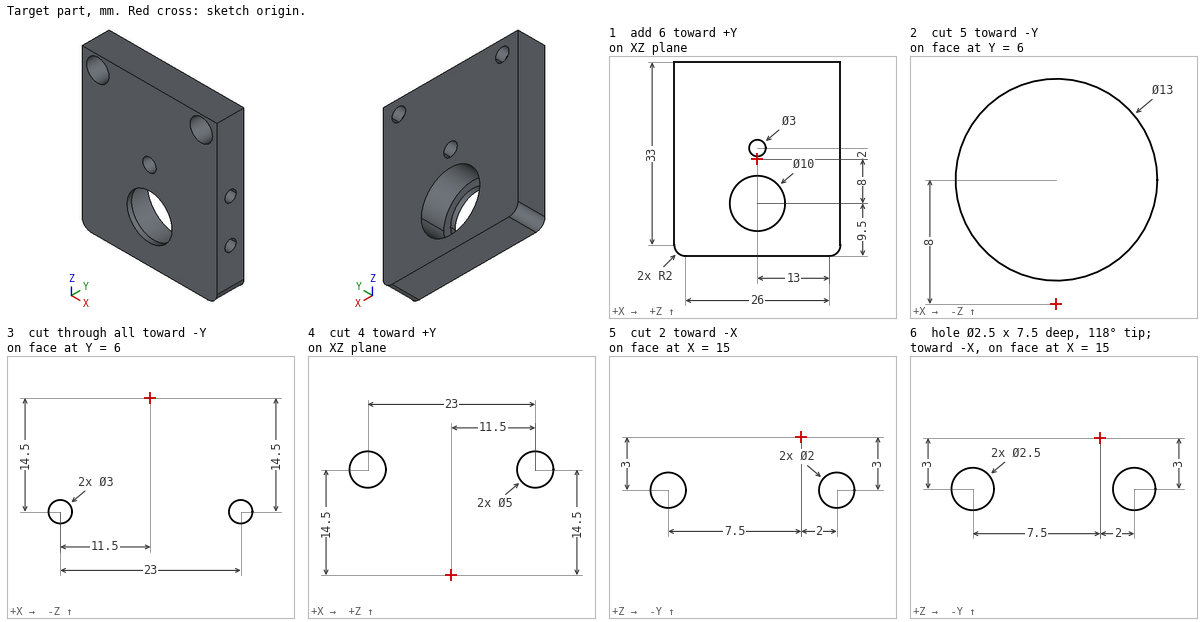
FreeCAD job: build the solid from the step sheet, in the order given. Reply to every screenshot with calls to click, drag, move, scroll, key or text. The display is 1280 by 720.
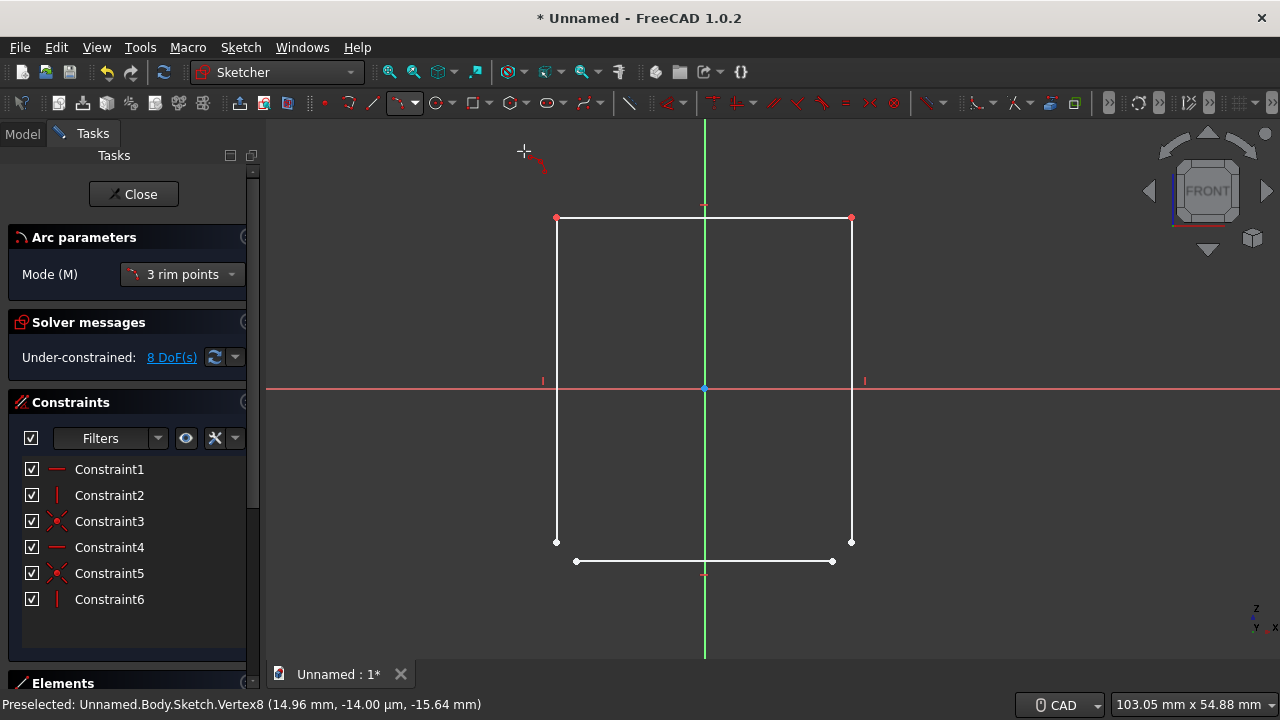
click(577, 561)
click(557, 542)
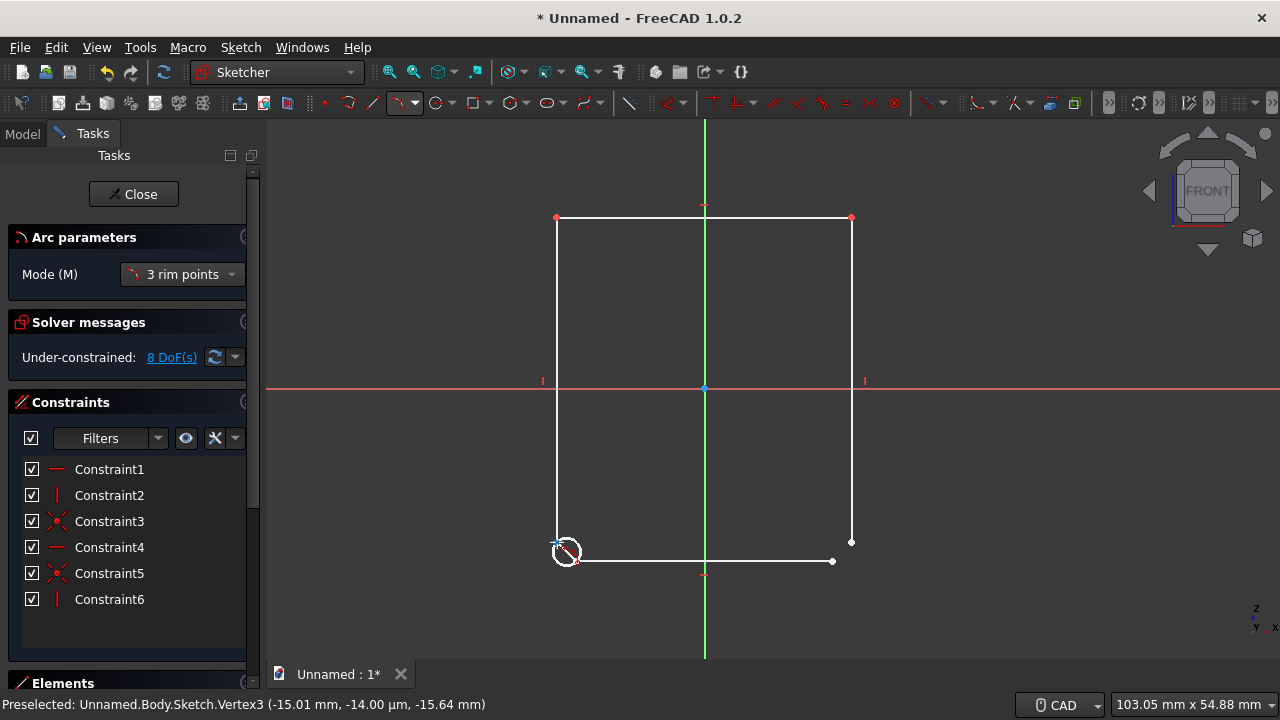
scroll(563, 555, up, 6)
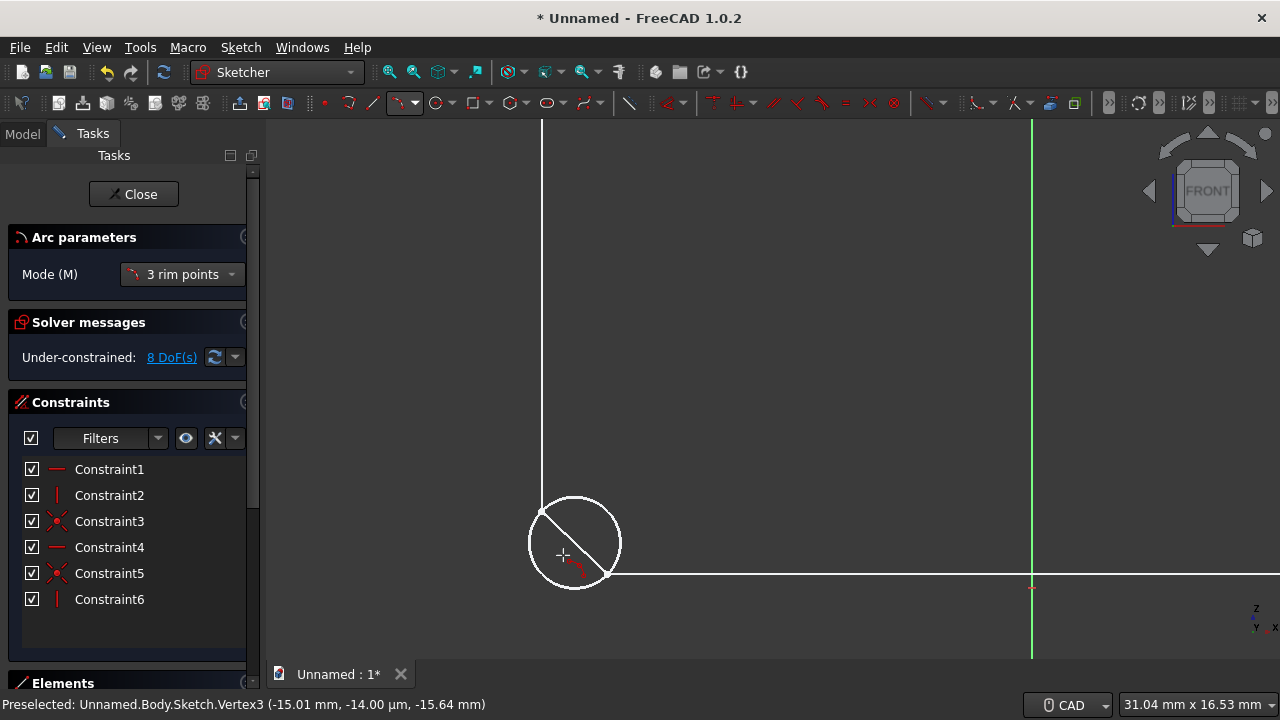
click(561, 553)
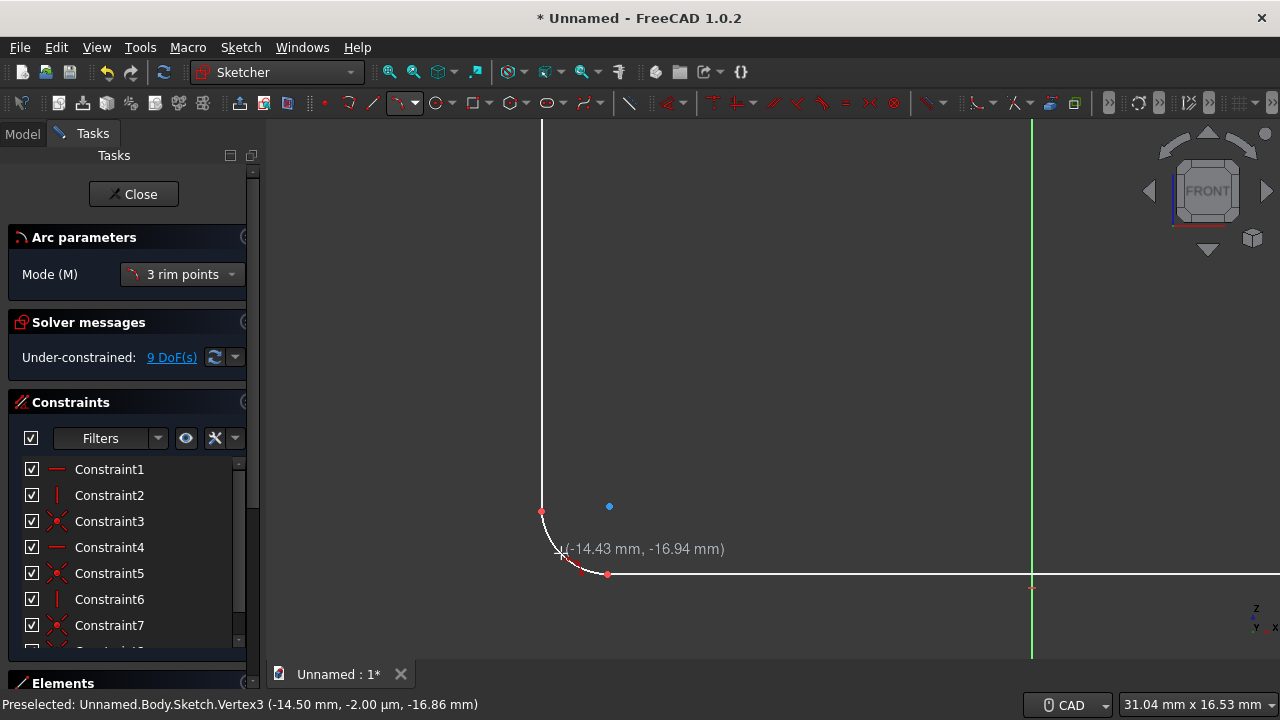
scroll(563, 556, down, 6)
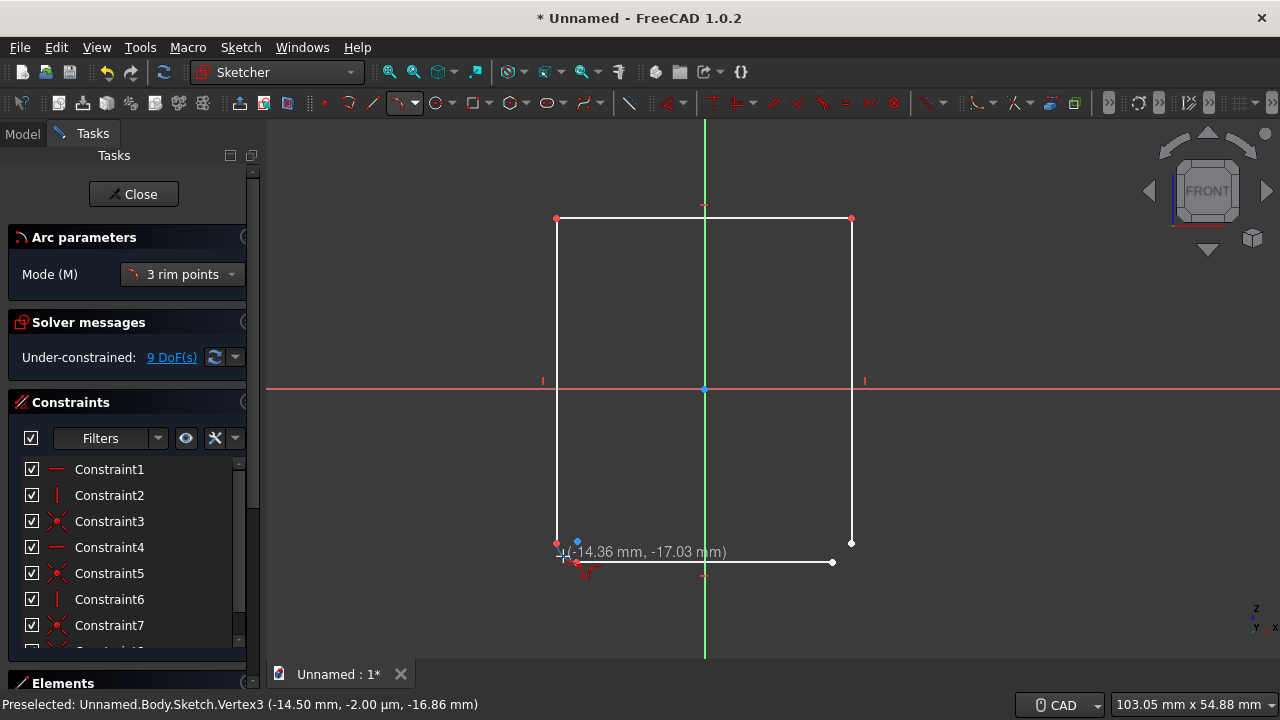
click(852, 543)
click(833, 562)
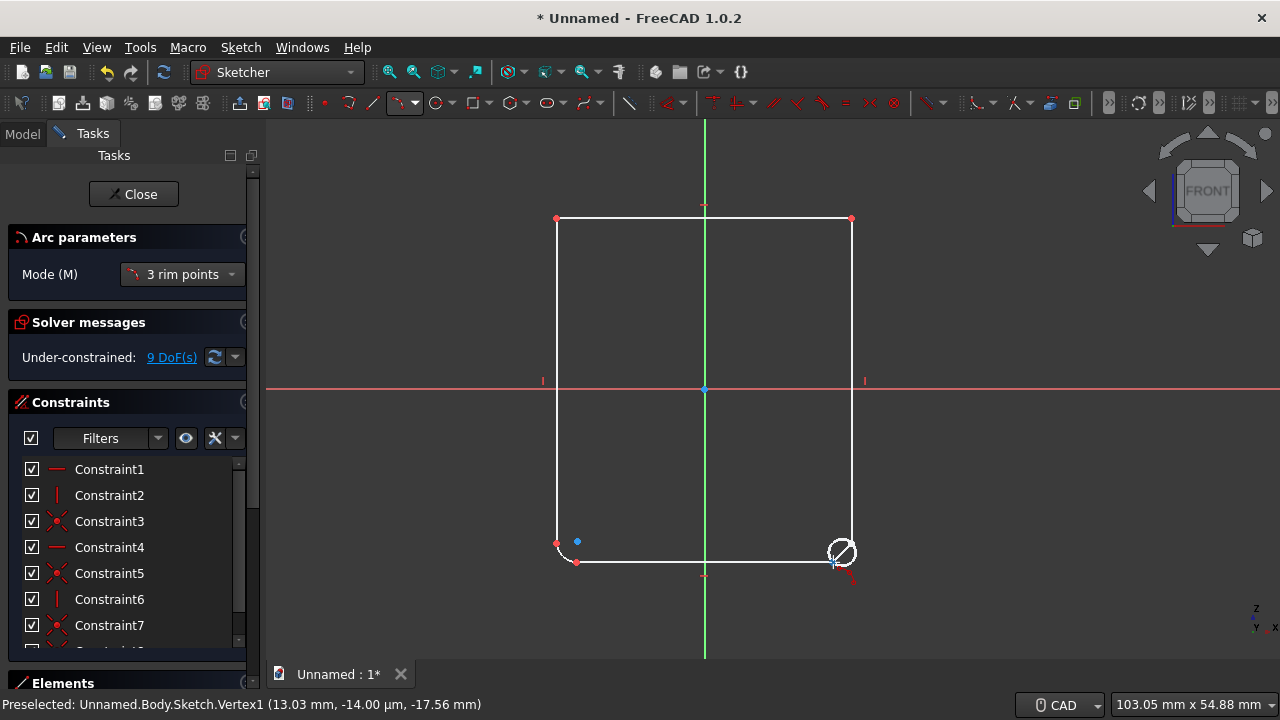
scroll(846, 556, up, 6)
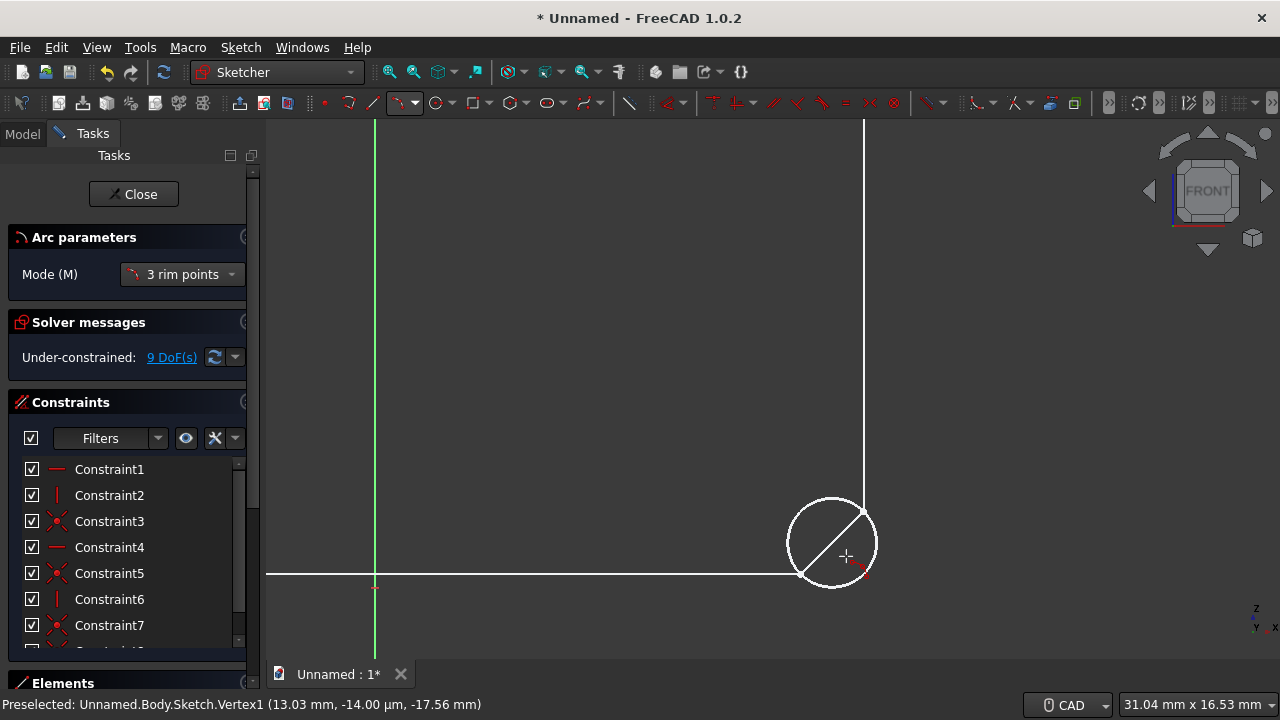
click(846, 553)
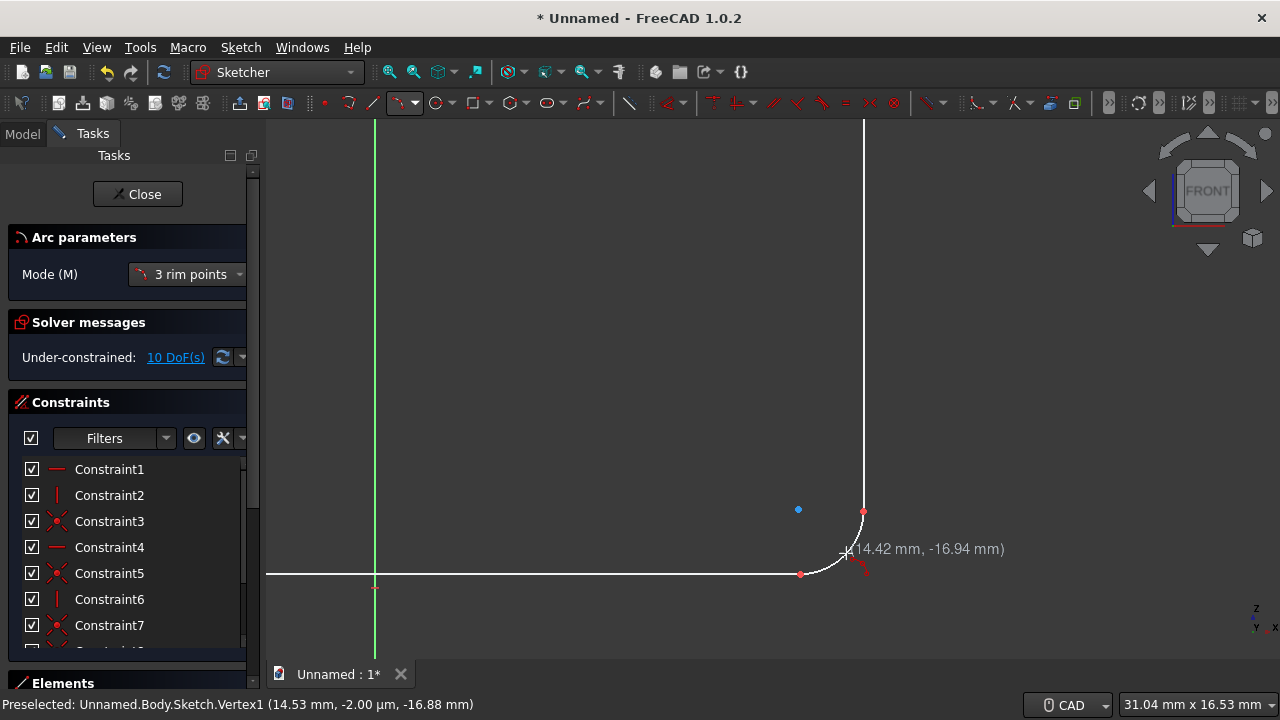
key(g)
key(c)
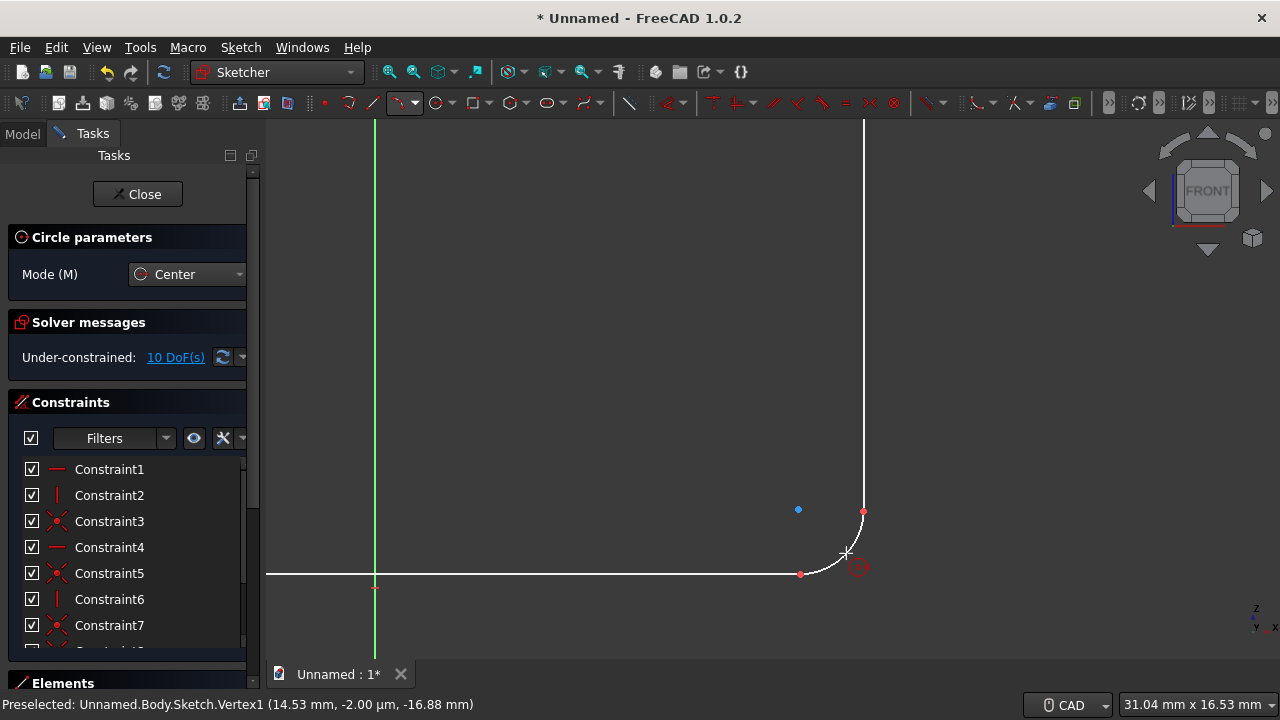
scroll(847, 556, down, 6)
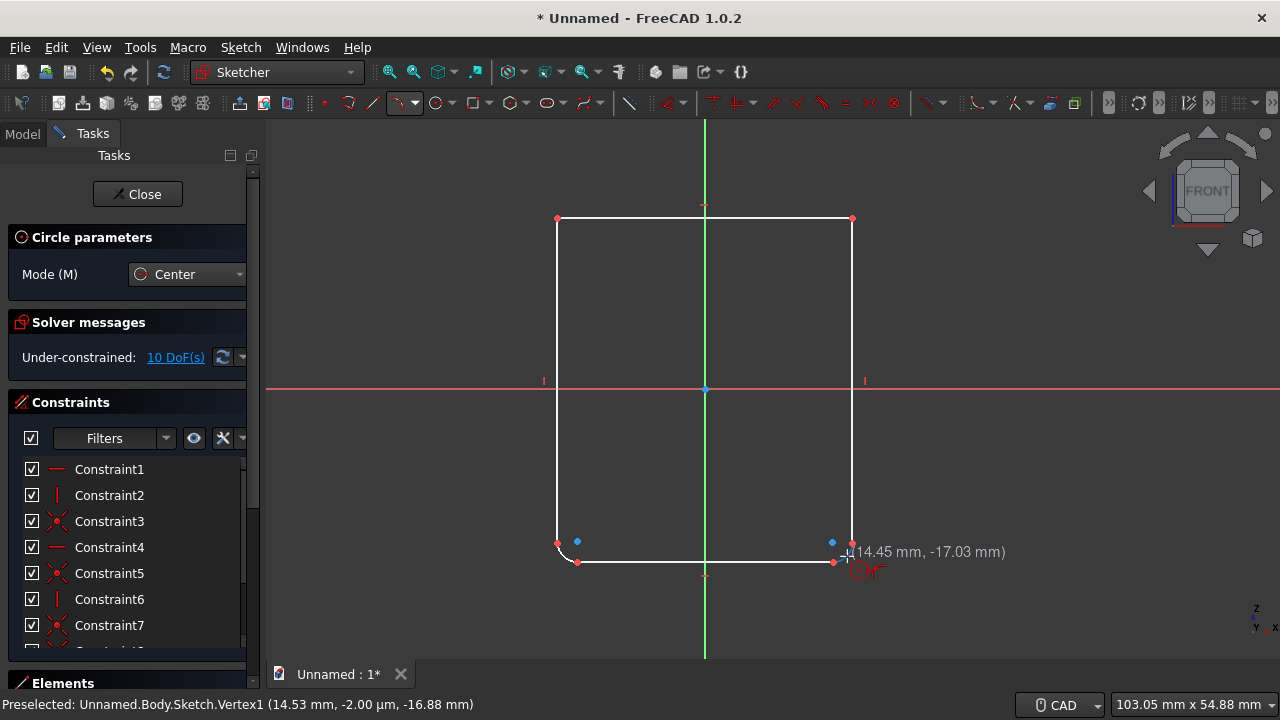
scroll(705, 370, up, 3)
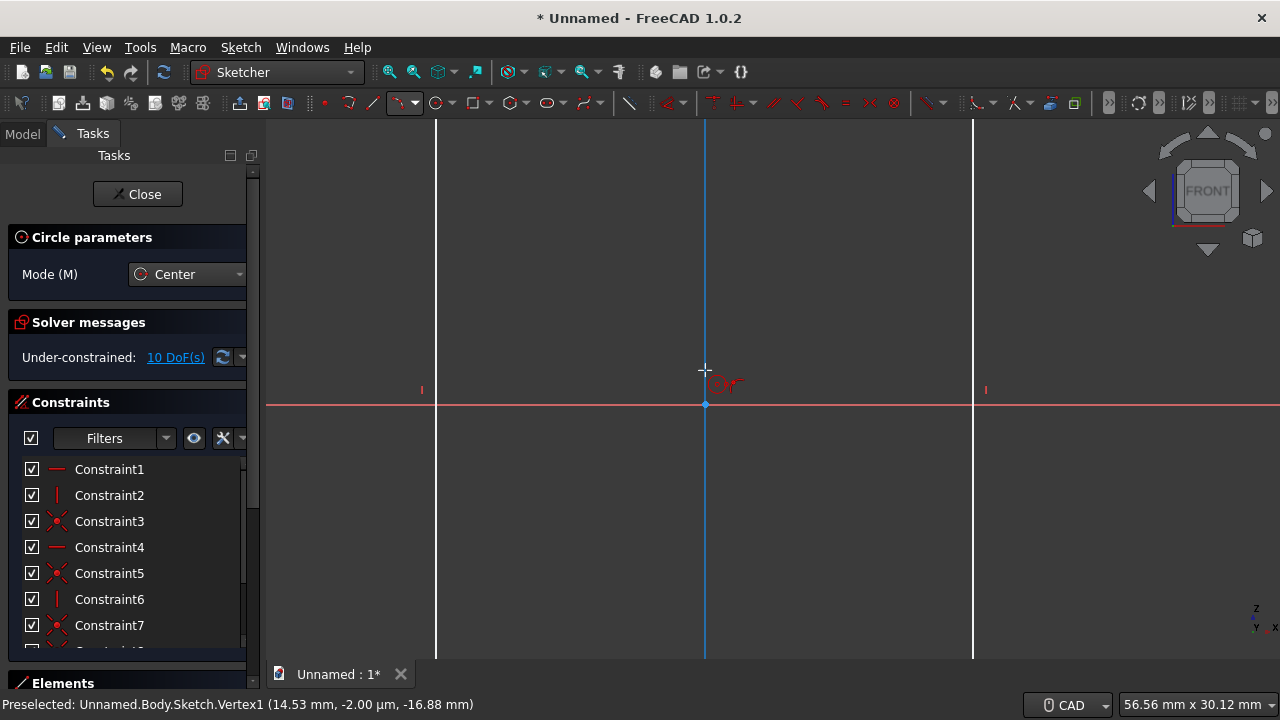
click(705, 369)
click(724, 350)